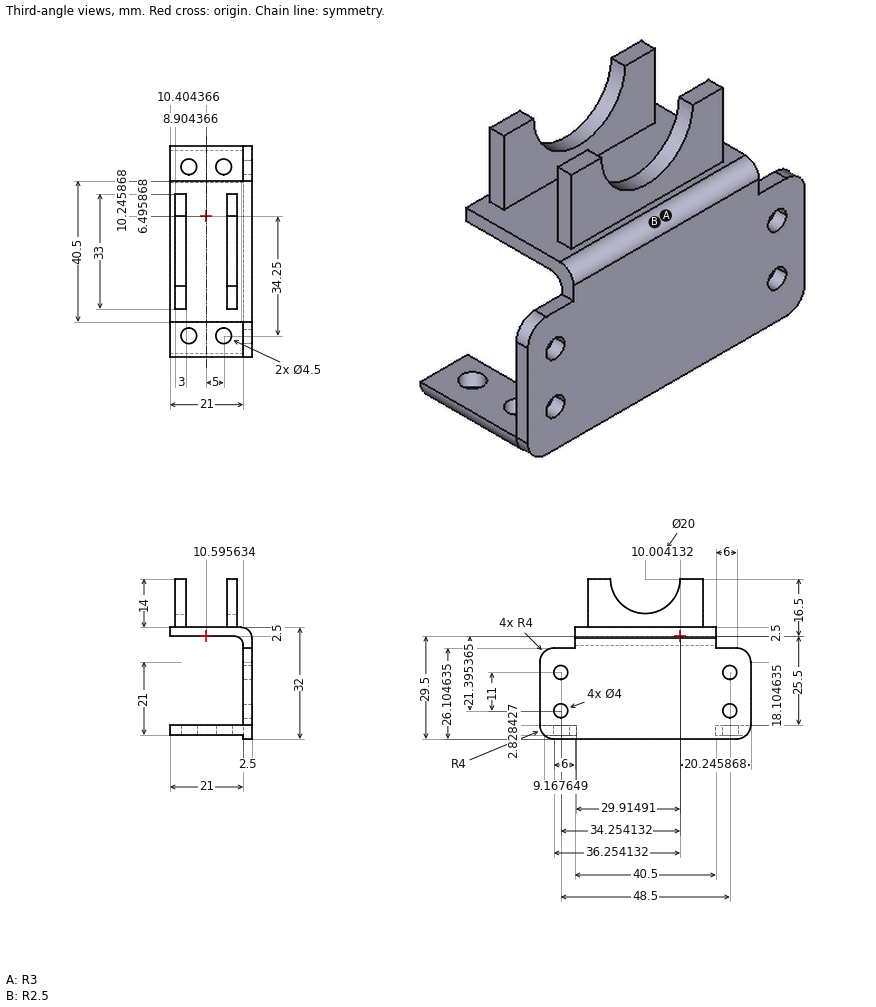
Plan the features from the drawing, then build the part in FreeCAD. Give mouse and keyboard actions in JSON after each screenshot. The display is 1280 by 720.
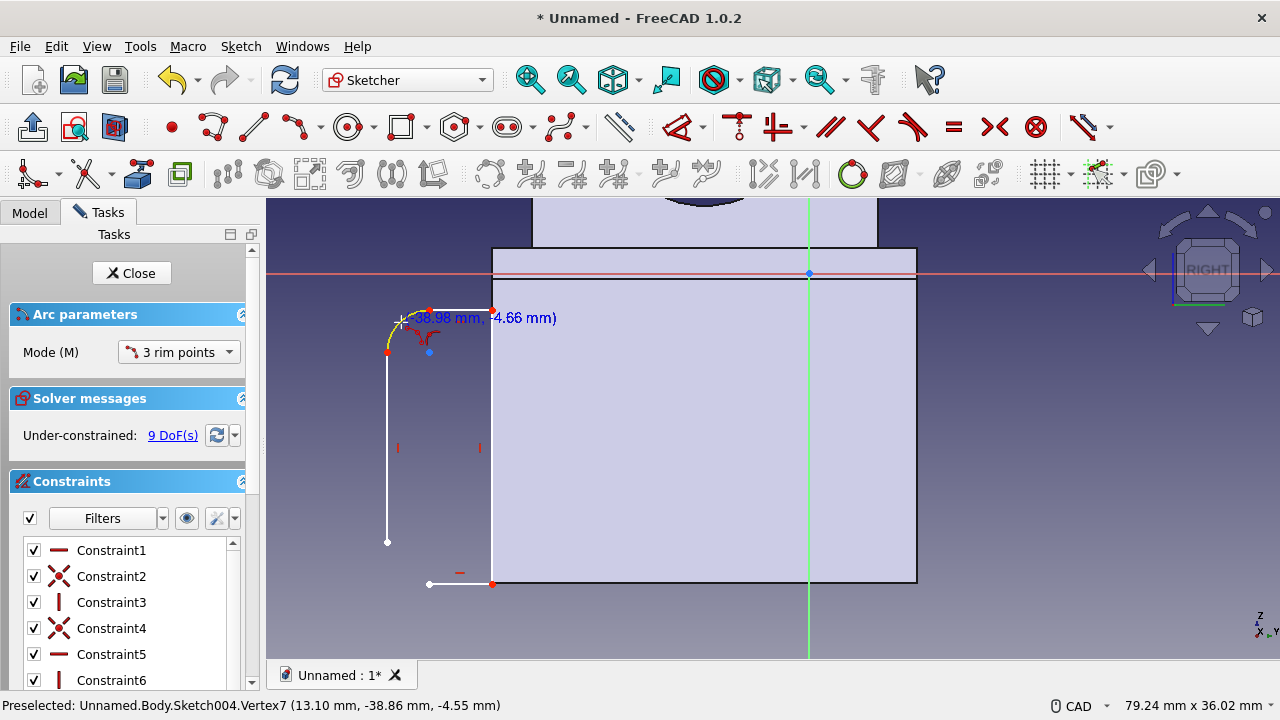
{"action": "left_click", "coordinate": [387, 542]}
{"action": "left_click", "coordinate": [429, 584]}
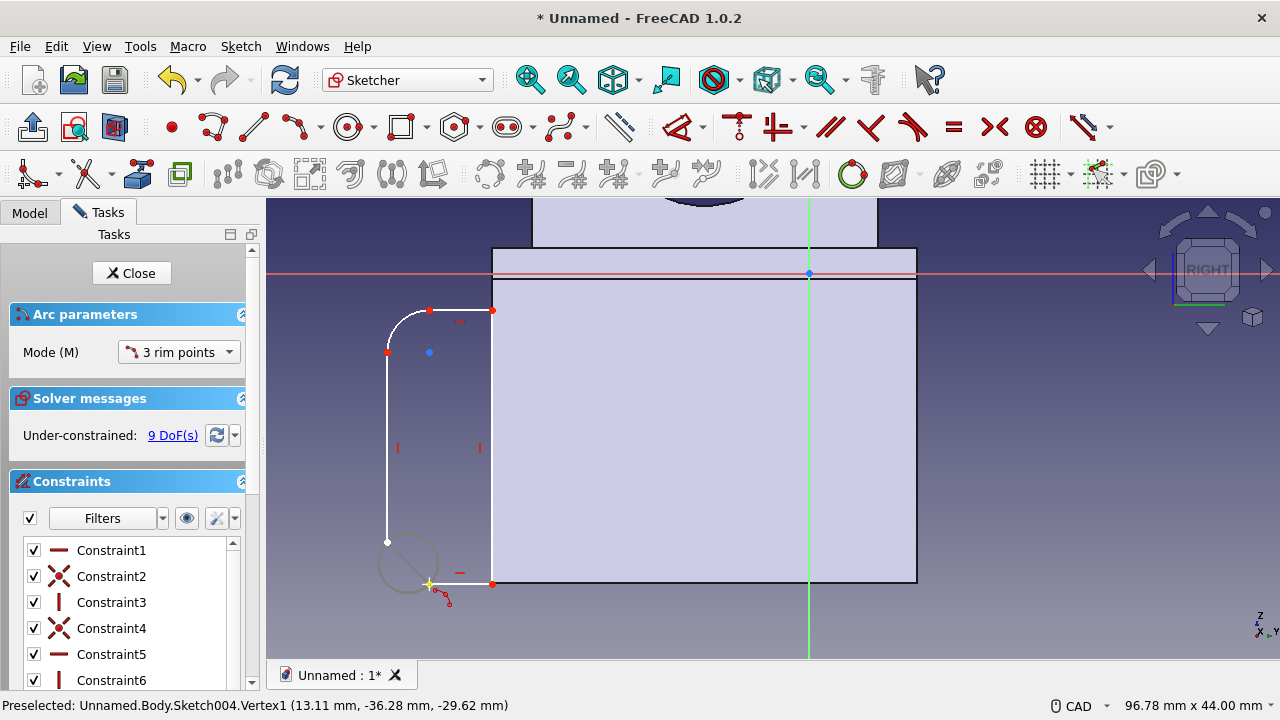
{"action": "scroll", "coordinate": [400, 571], "scroll_direction": "up", "scroll_amount": 2}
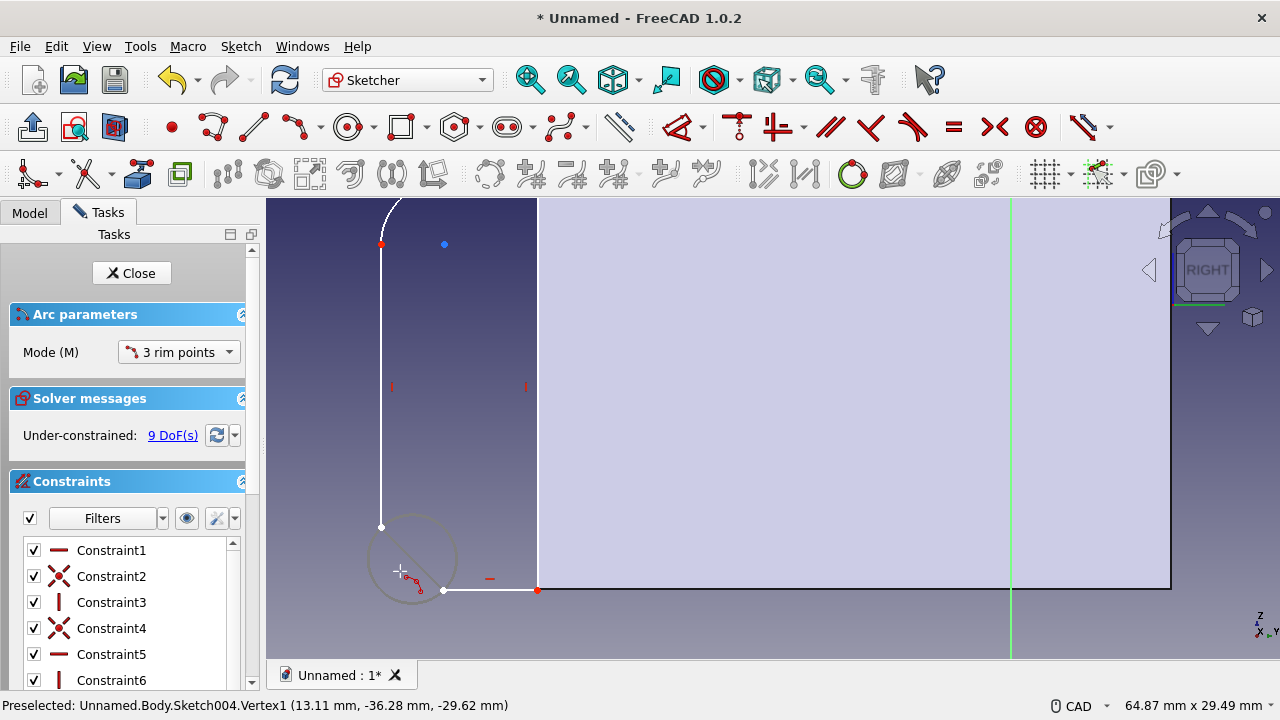
{"action": "left_click", "coordinate": [400, 570]}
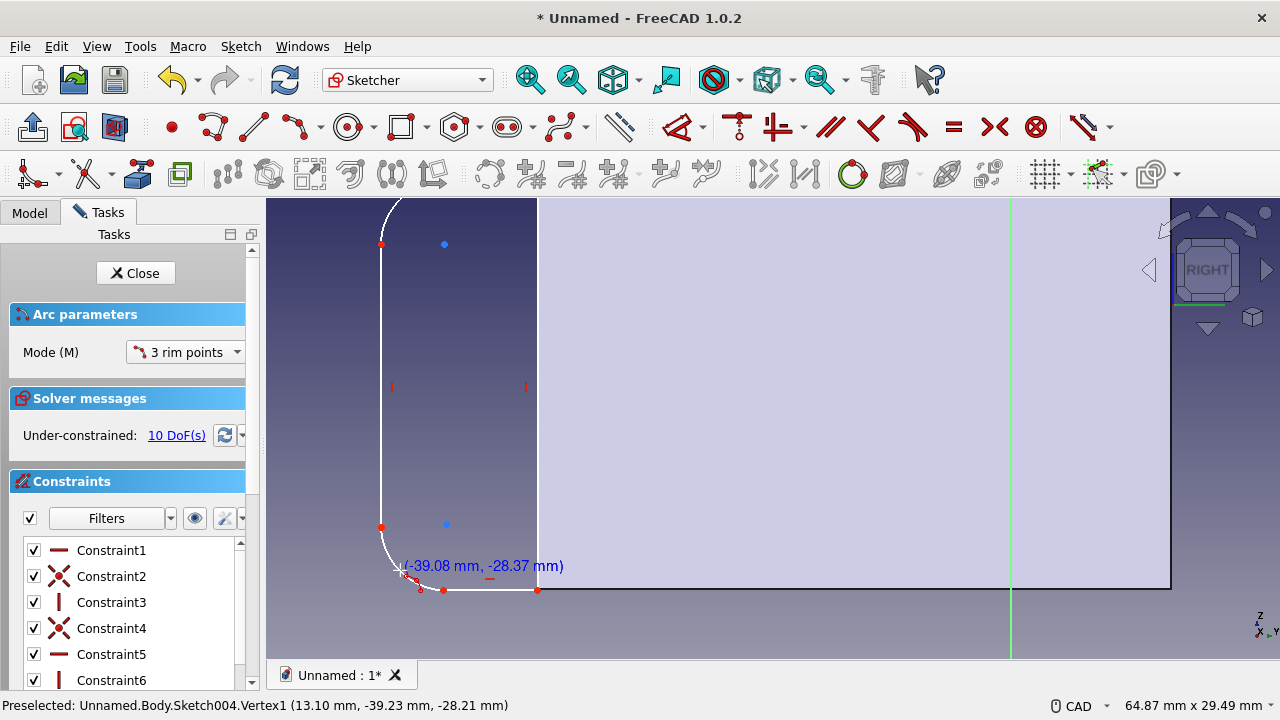
{"action": "left_click", "coordinate": [254, 128]}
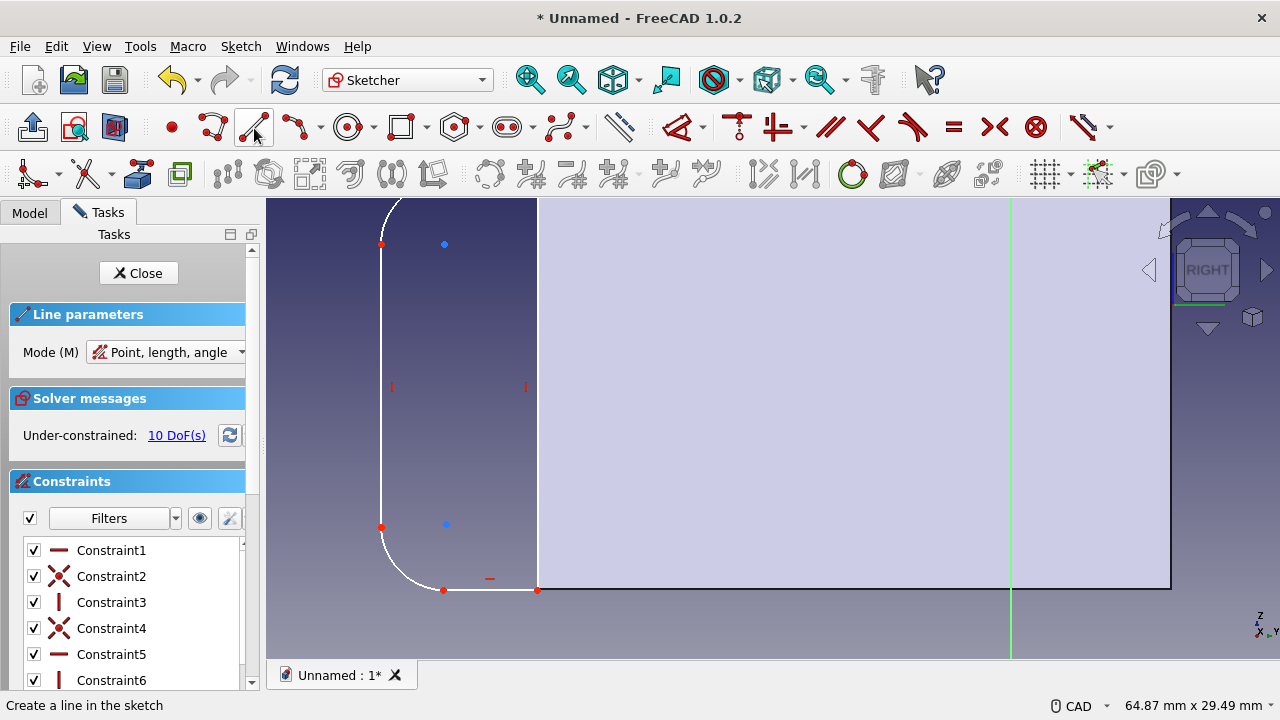
{"action": "scroll", "coordinate": [400, 572], "scroll_direction": "down", "scroll_amount": 2}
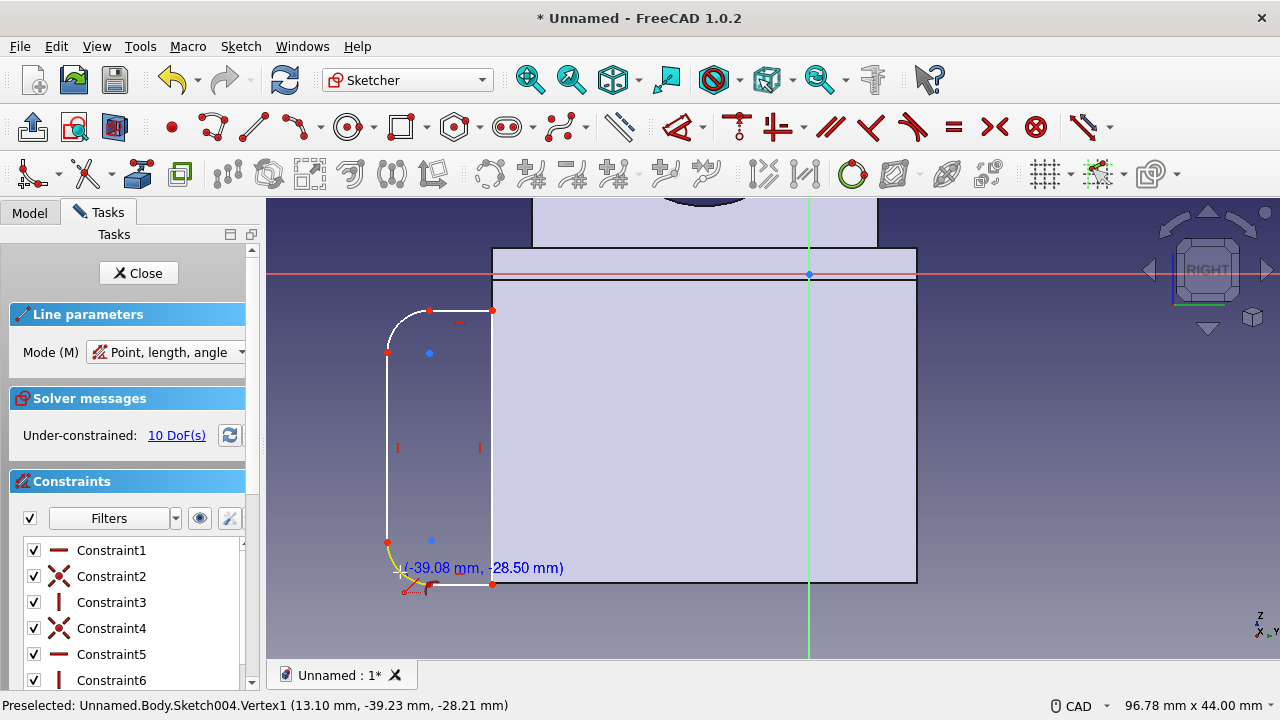
{"action": "left_click", "coordinate": [1022, 541]}
{"action": "left_click", "coordinate": [1022, 352]}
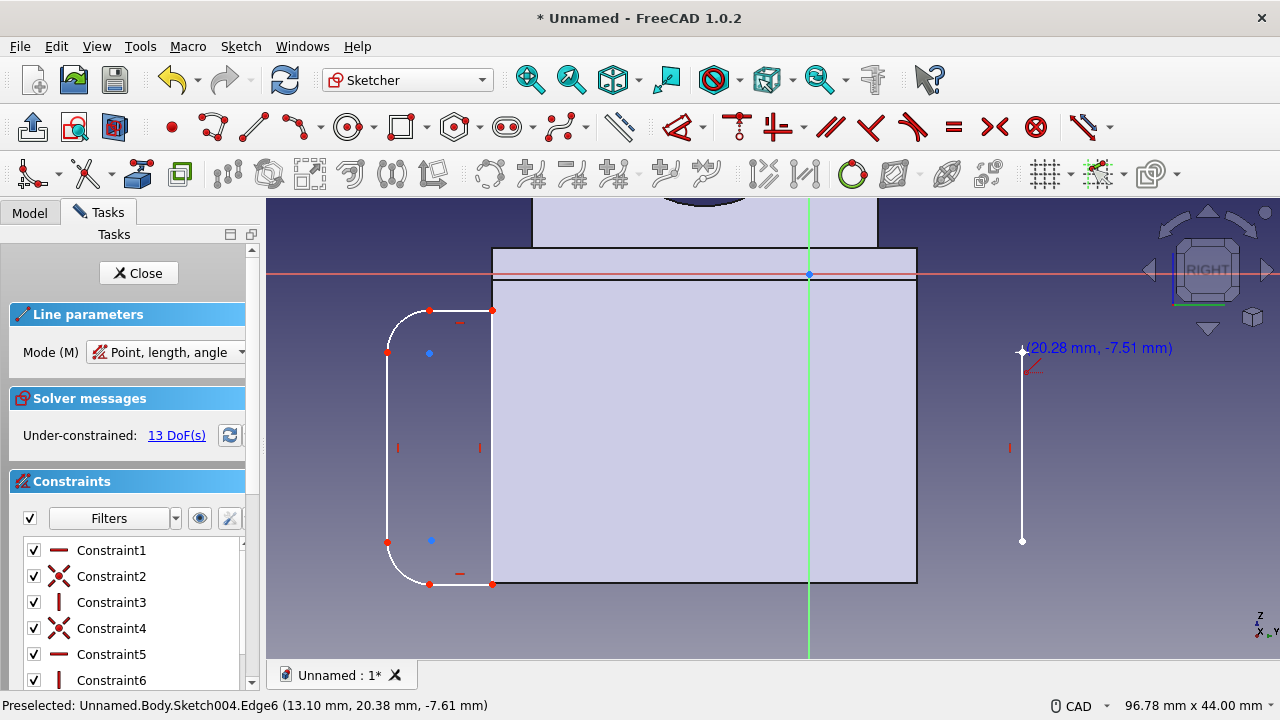
{"action": "left_click", "coordinate": [213, 128]}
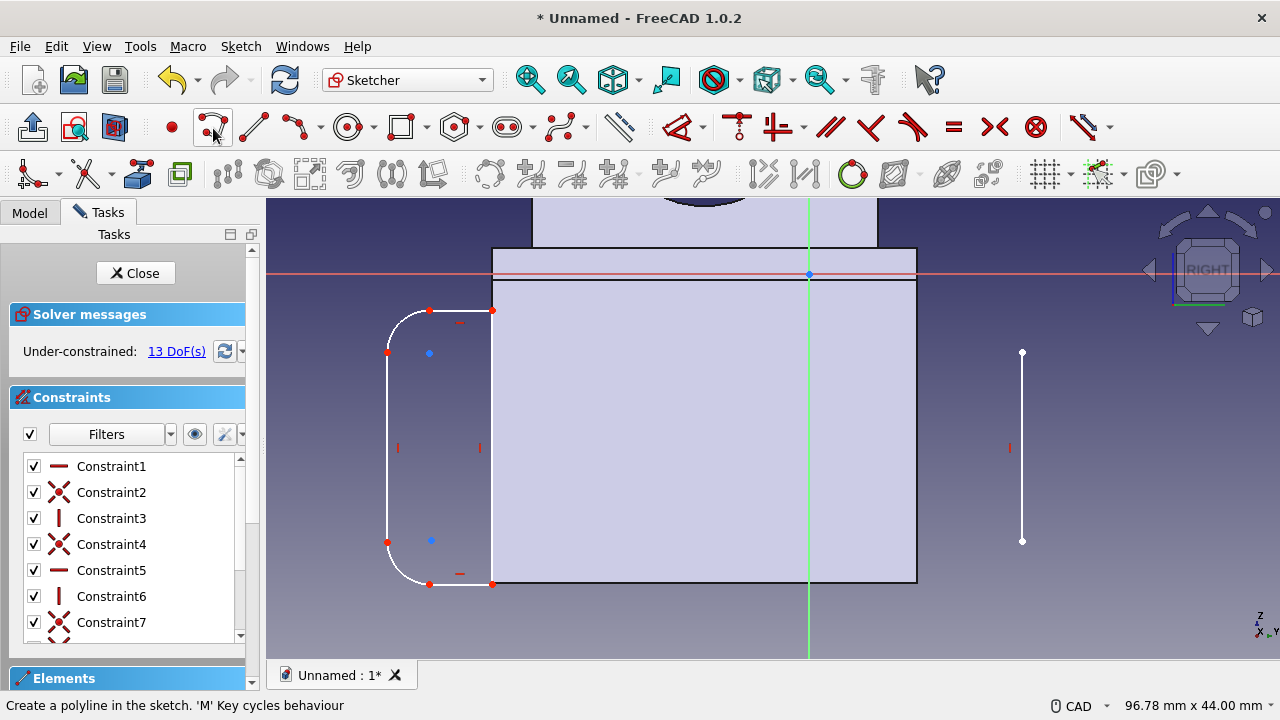
{"action": "left_click", "coordinate": [980, 310]}
{"action": "left_click", "coordinate": [917, 310]}
{"action": "left_click", "coordinate": [917, 583]}
{"action": "left_click", "coordinate": [980, 583]}
{"action": "right_click", "coordinate": [980, 583]}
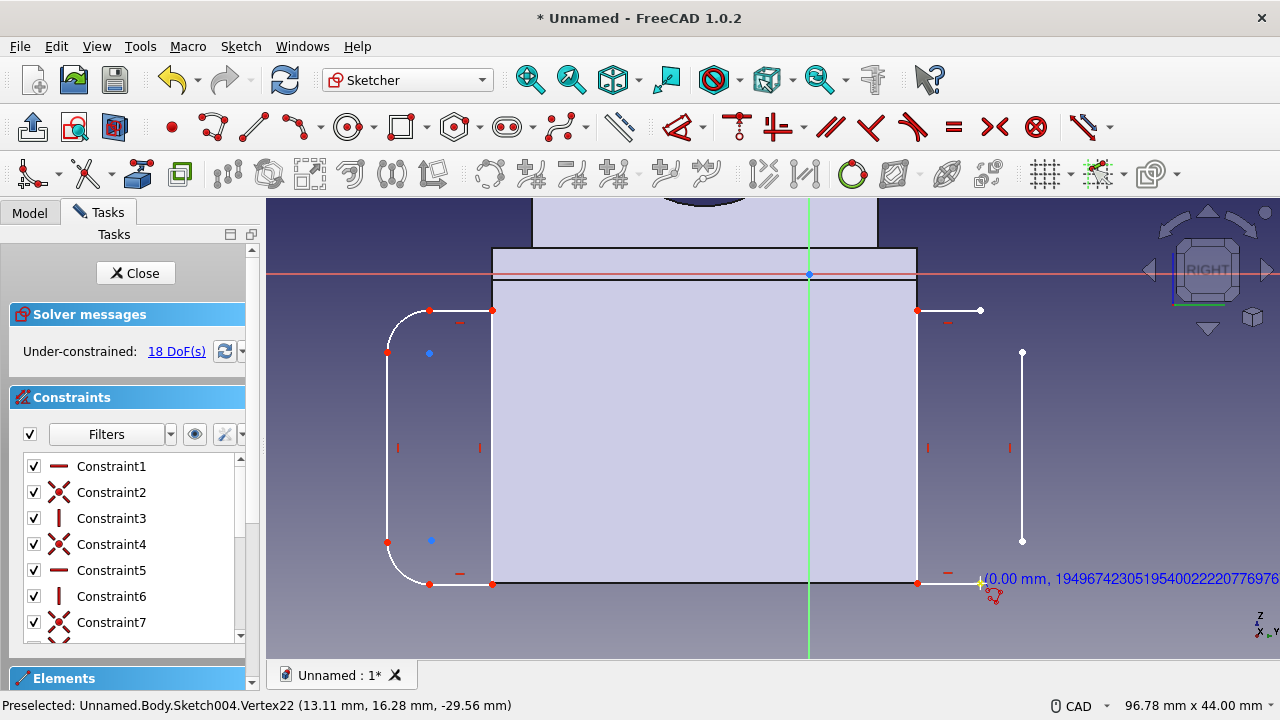
{"action": "left_click", "coordinate": [294, 128]}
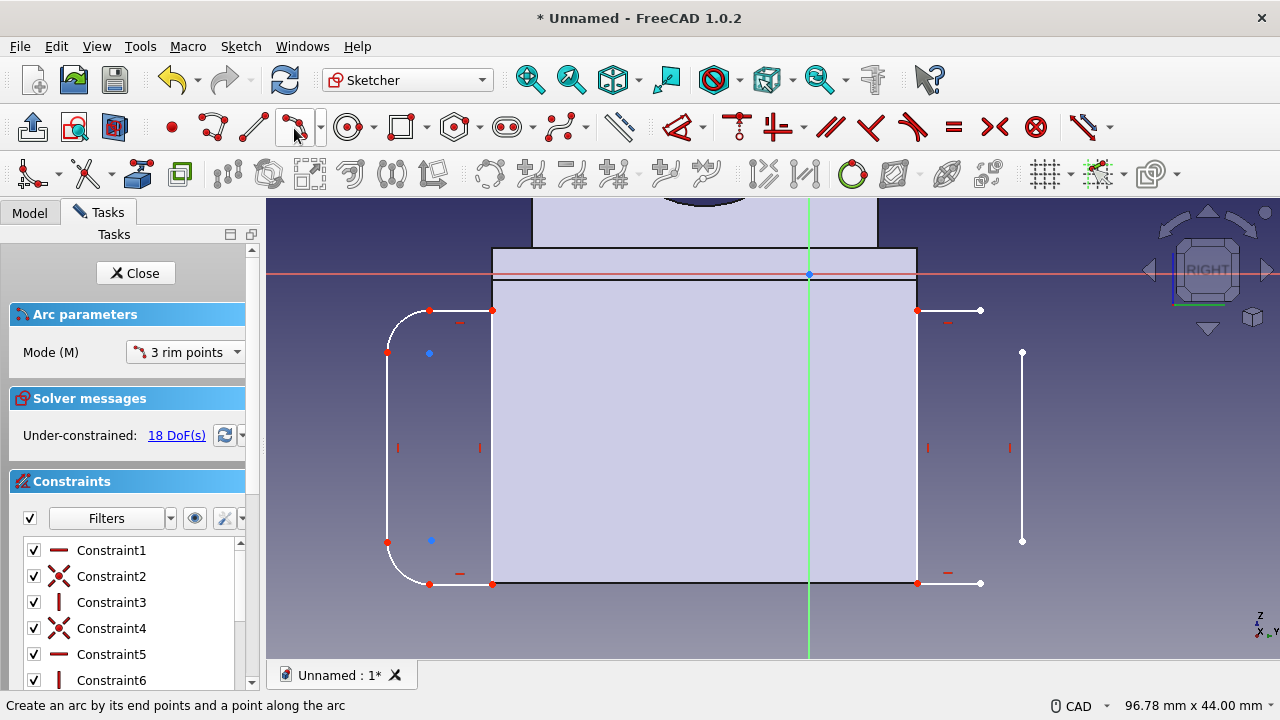
{"action": "left_click", "coordinate": [1022, 353]}
{"action": "left_click", "coordinate": [980, 311]}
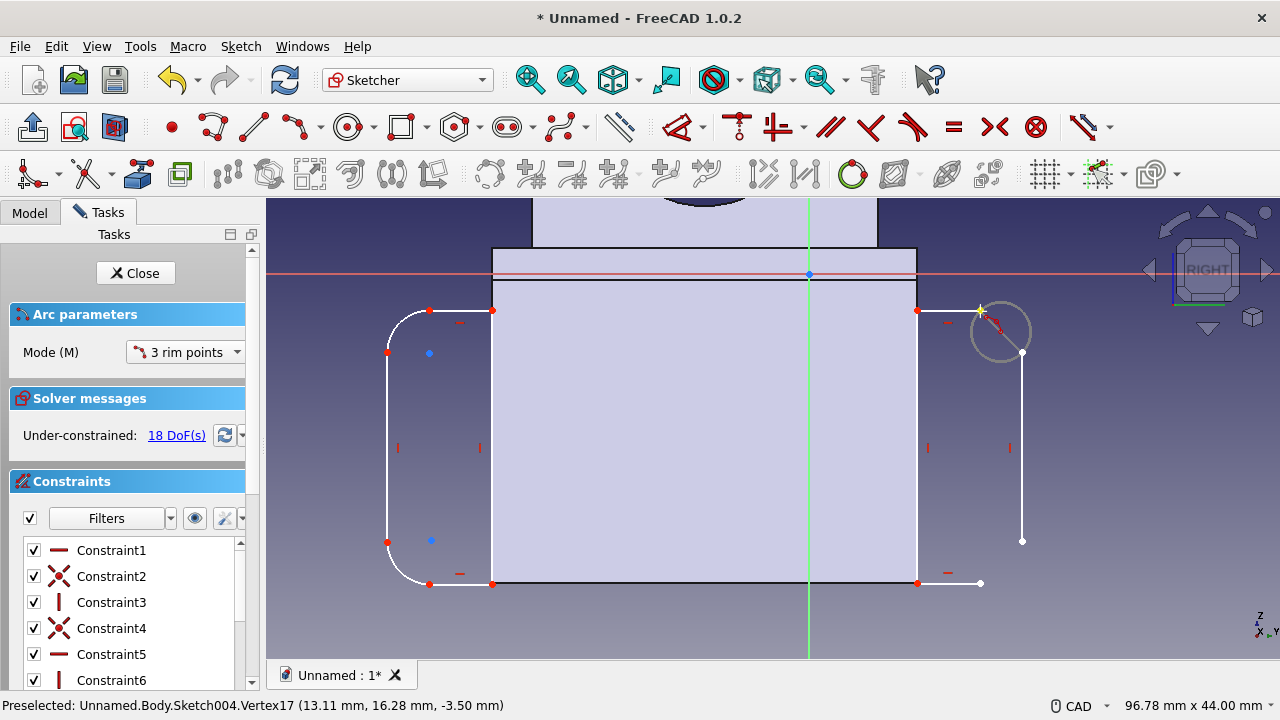
{"action": "scroll", "coordinate": [1009, 322], "scroll_direction": "up", "scroll_amount": 2}